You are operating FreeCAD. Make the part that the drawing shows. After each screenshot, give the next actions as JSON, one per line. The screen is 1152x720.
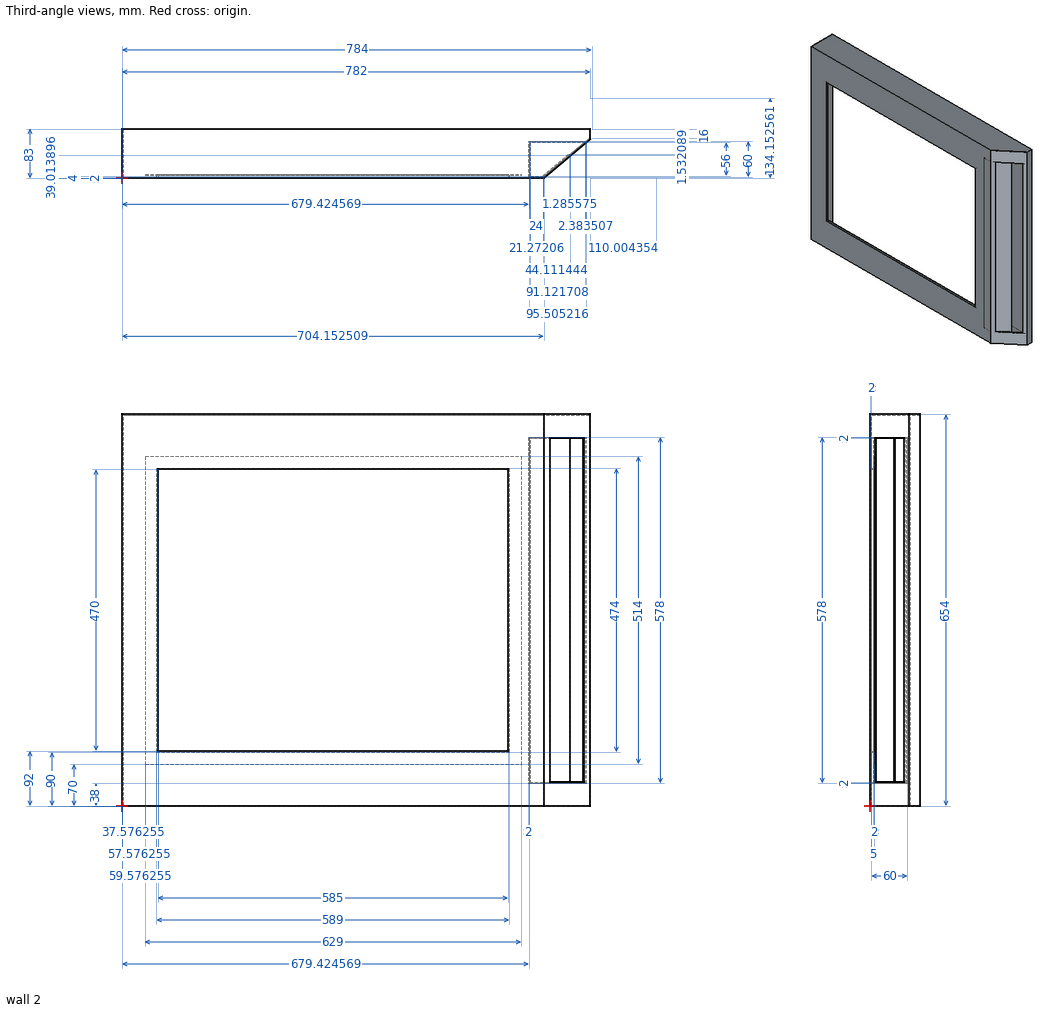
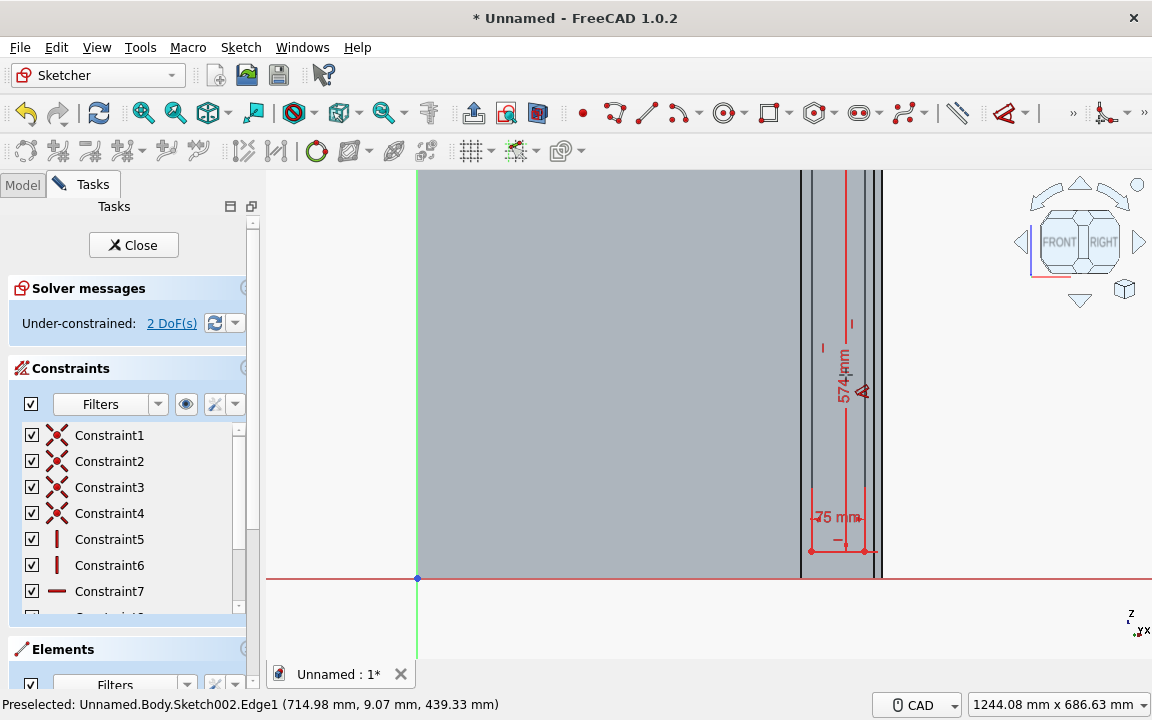
{"action": "scroll", "coordinate": [812, 552], "scroll_direction": "up", "scroll_amount": 2}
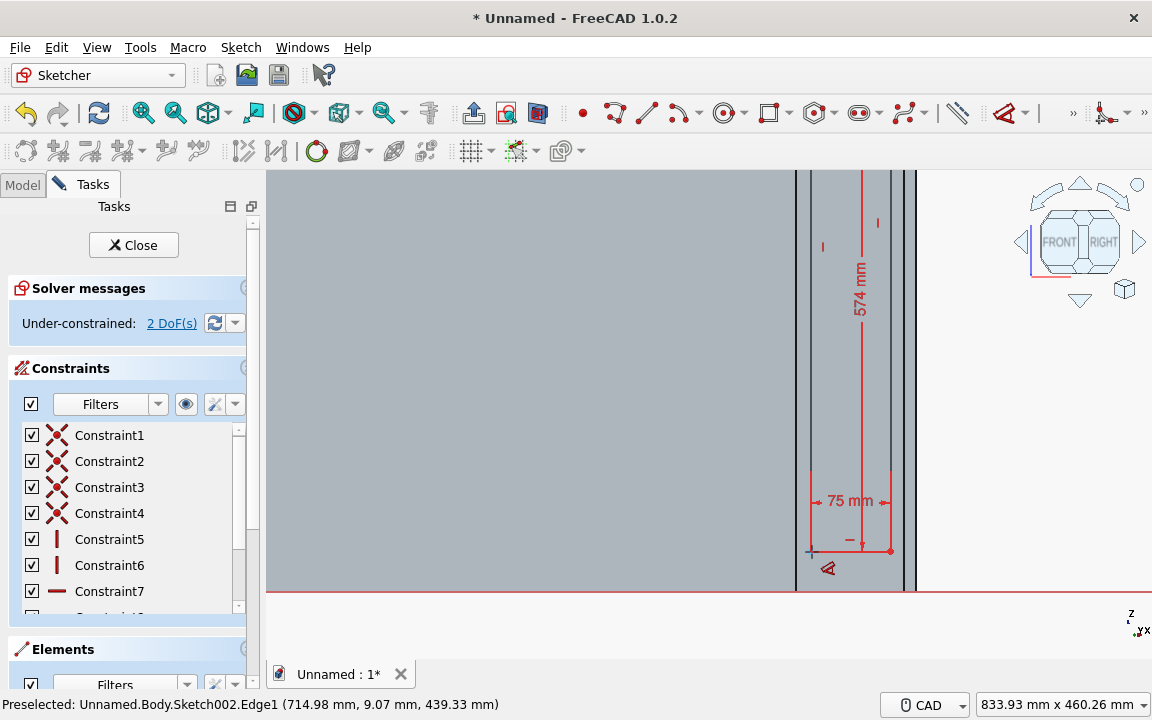
{"action": "left_click", "coordinate": [811, 552]}
{"action": "left_click", "coordinate": [845, 572]}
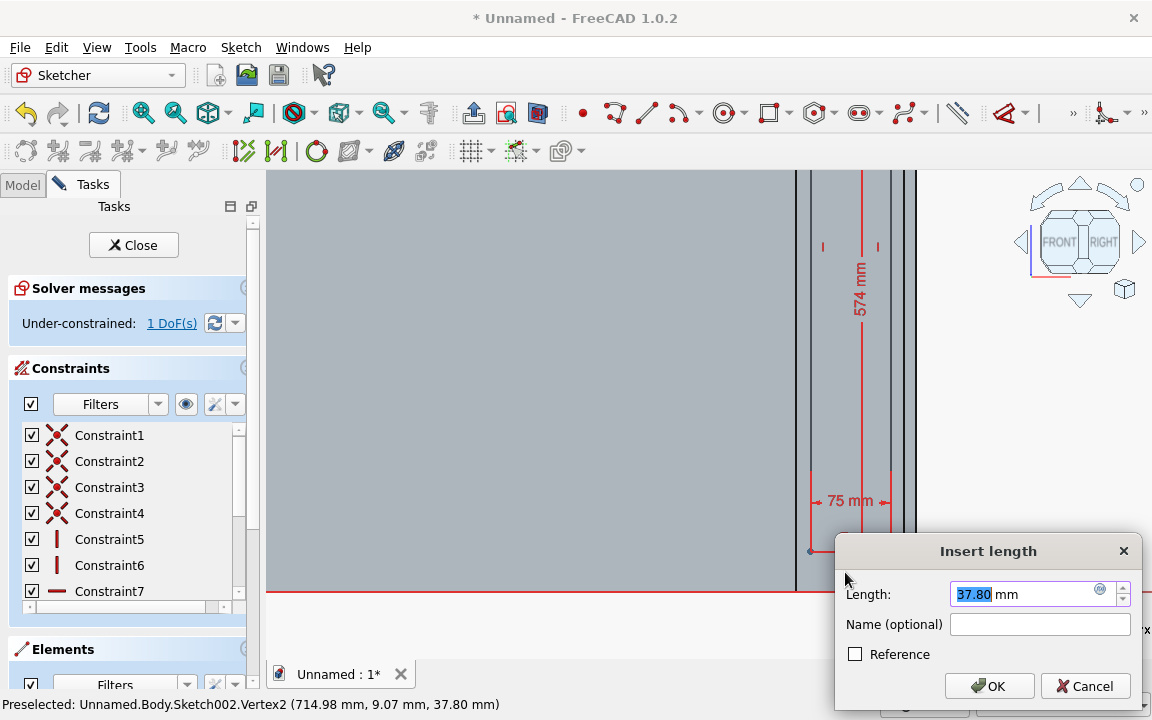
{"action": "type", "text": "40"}
{"action": "key", "text": "Return"}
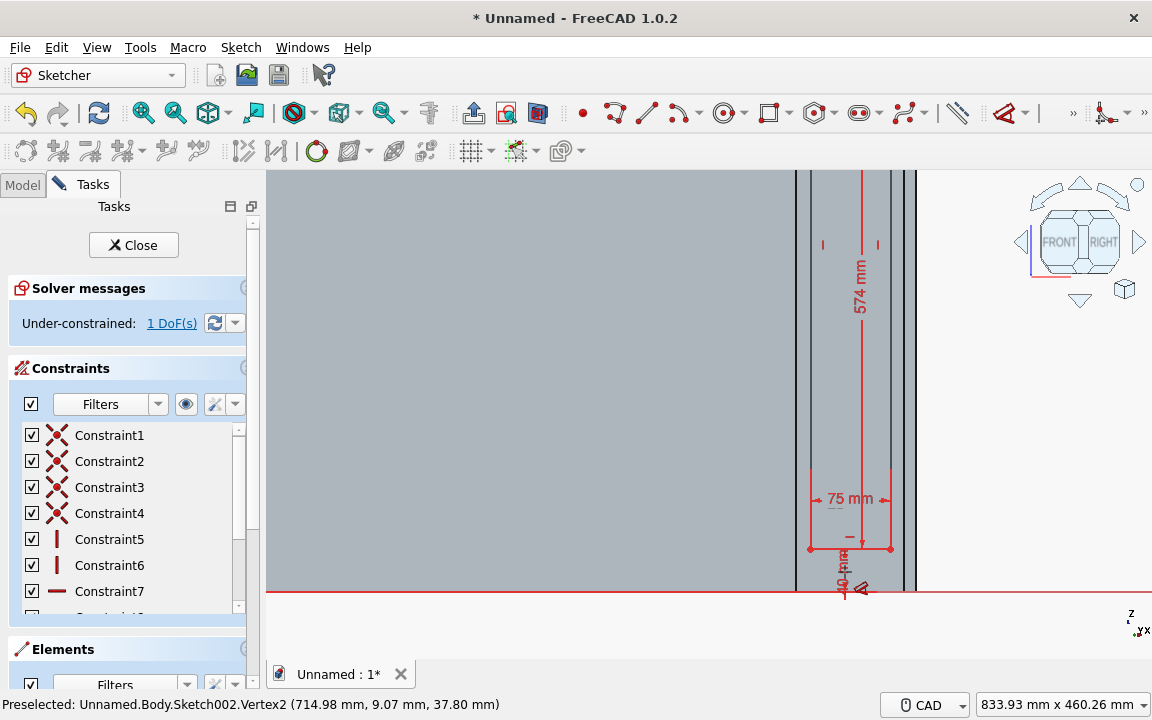
{"action": "scroll", "coordinate": [709, 536], "scroll_direction": "down", "scroll_amount": 4}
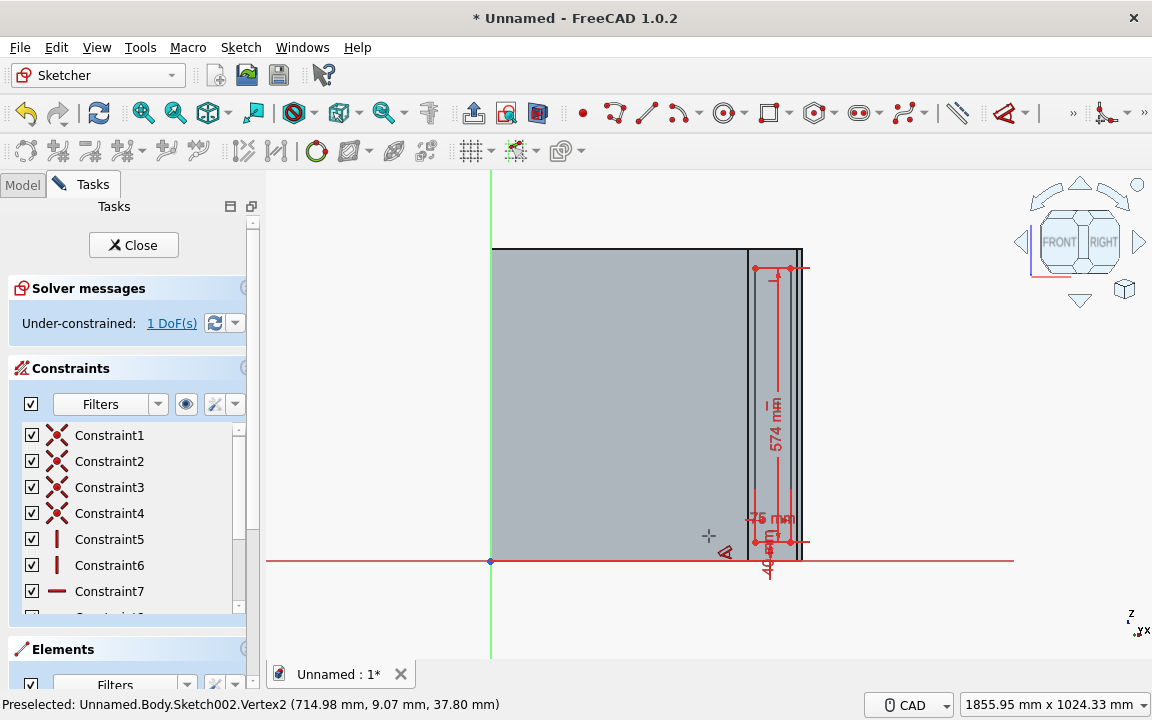
{"action": "left_click", "coordinate": [755, 268]}
{"action": "left_click", "coordinate": [623, 595]}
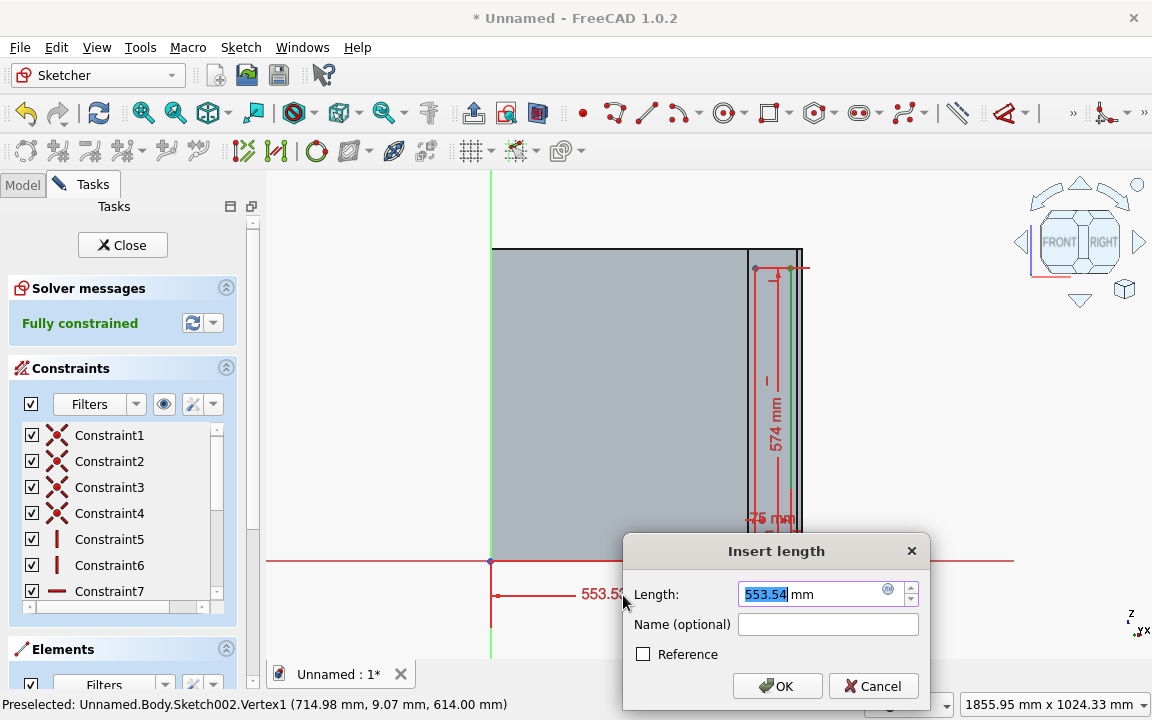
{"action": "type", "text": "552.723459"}
{"action": "key", "text": "Return"}
{"action": "key", "text": "Escape"}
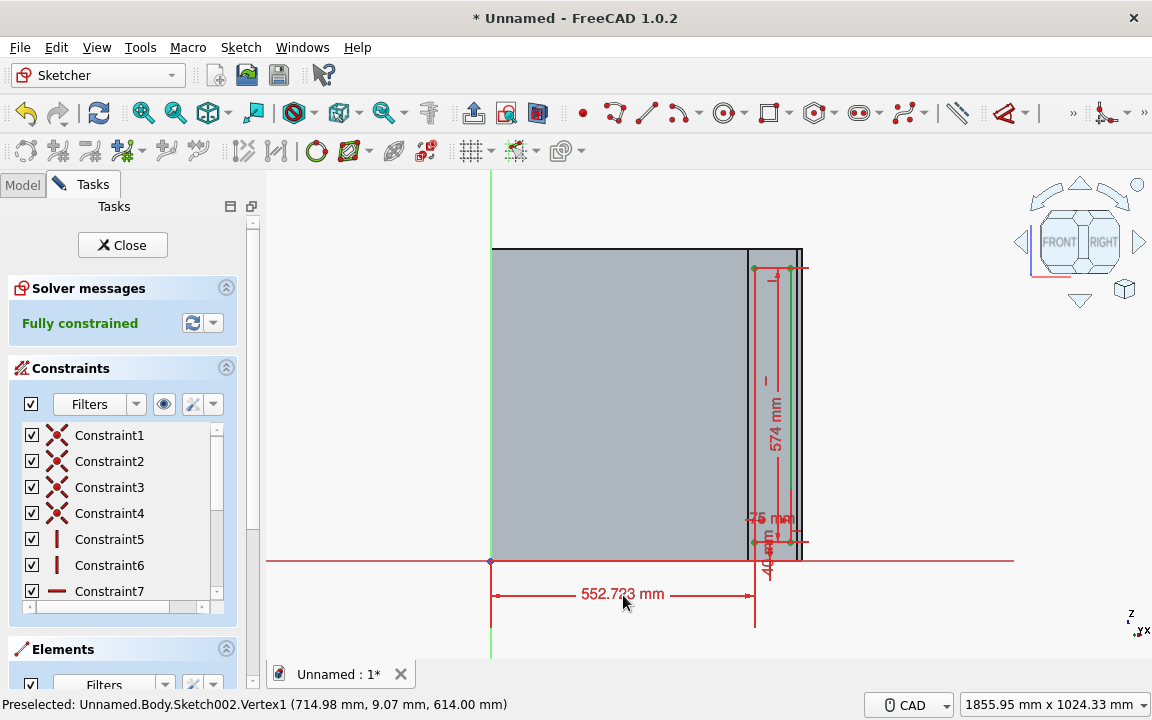
{"action": "left_click", "coordinate": [123, 245]}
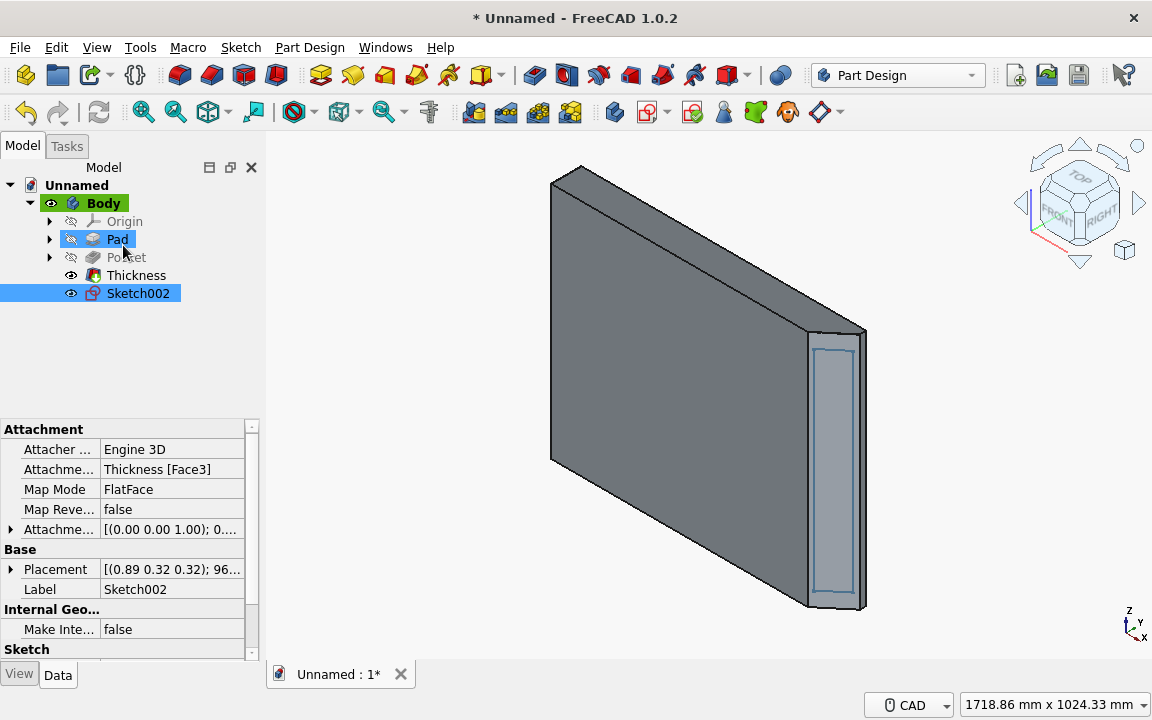
{"action": "left_click", "coordinate": [536, 76]}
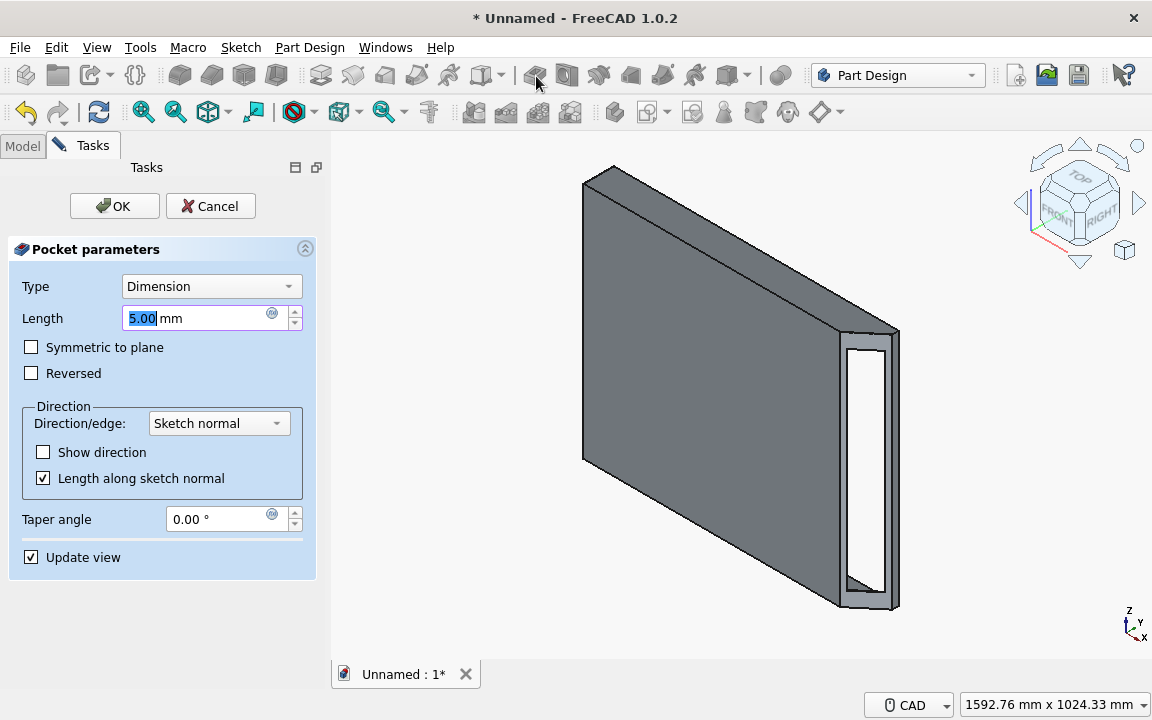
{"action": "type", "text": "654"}
{"action": "key", "text": "Tab"}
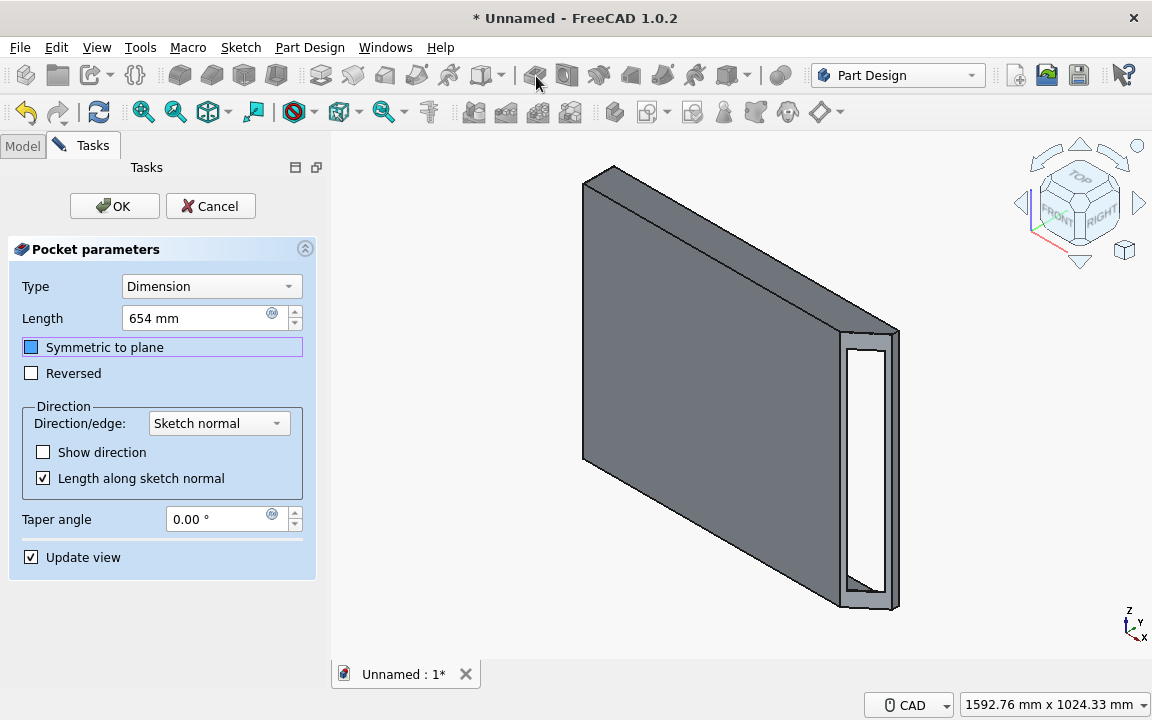
{"action": "left_click", "coordinate": [115, 206]}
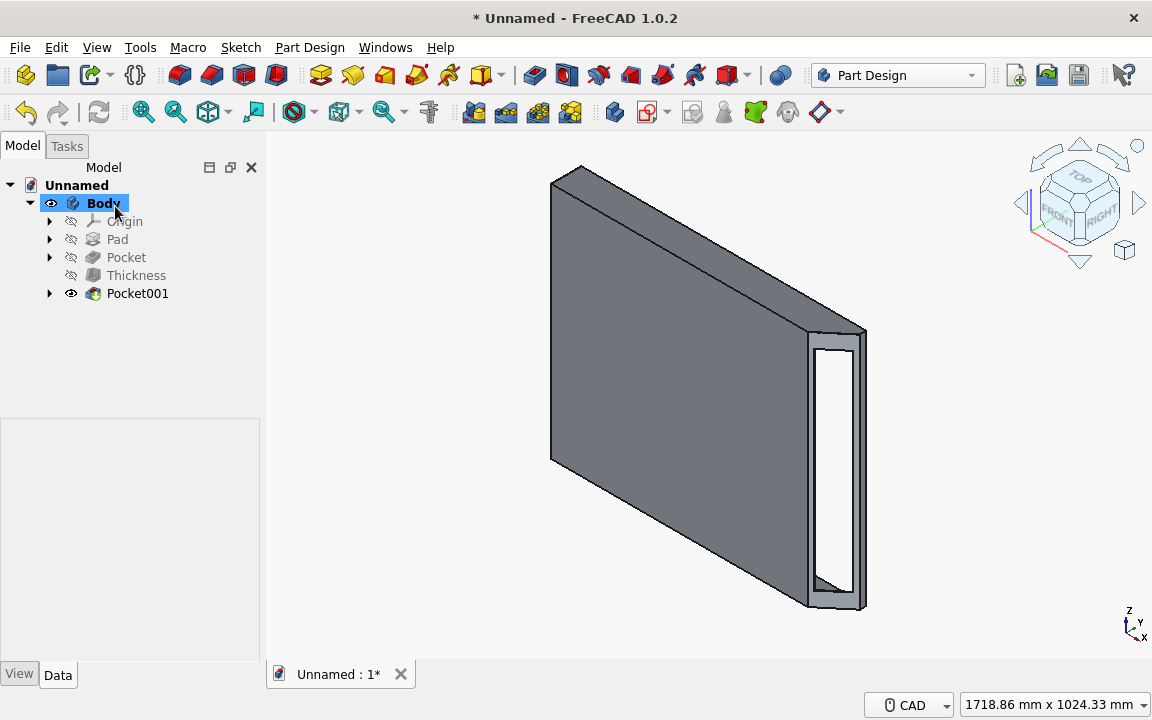
{"action": "key", "text": "4"}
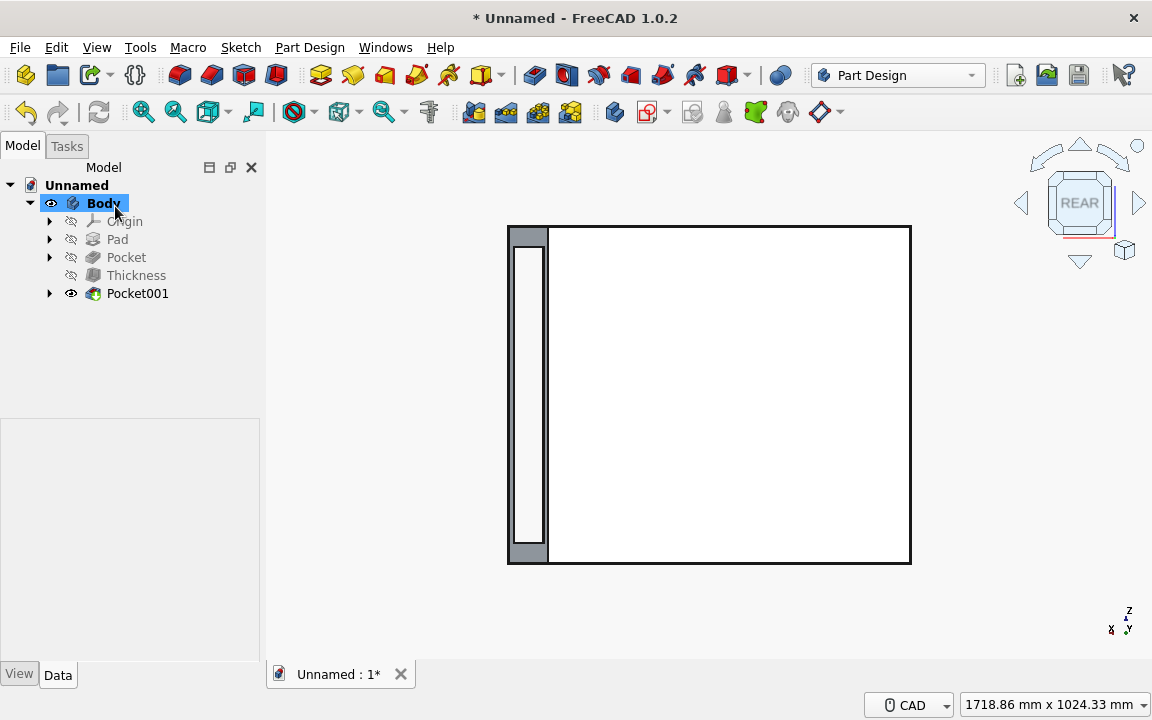
{"action": "left_click", "coordinate": [729, 394]}